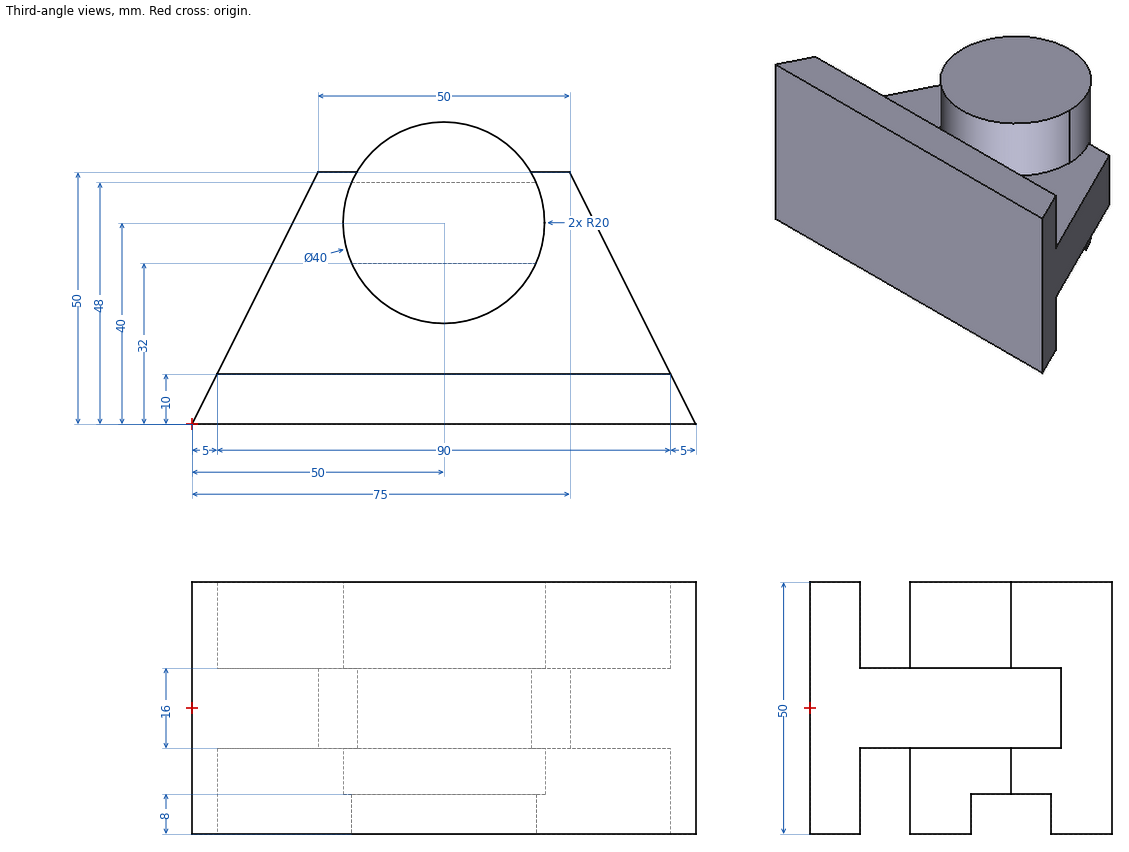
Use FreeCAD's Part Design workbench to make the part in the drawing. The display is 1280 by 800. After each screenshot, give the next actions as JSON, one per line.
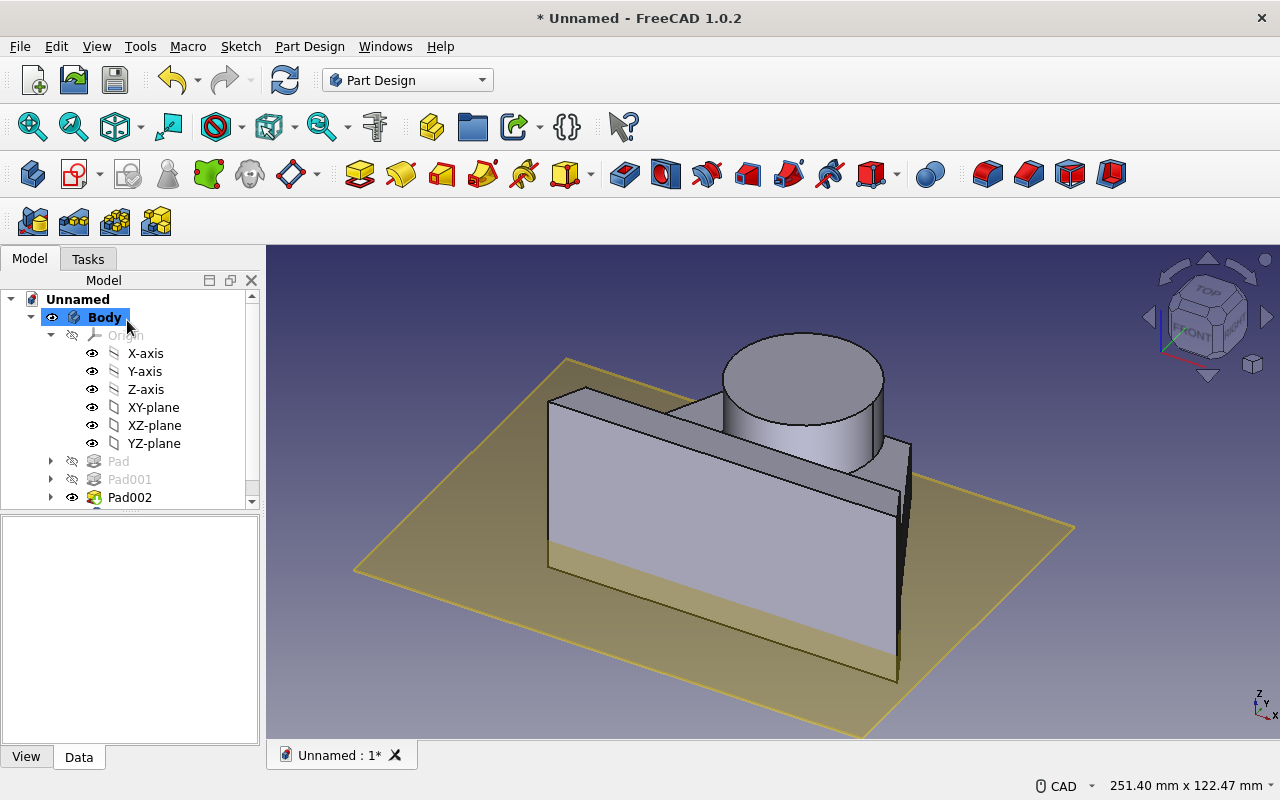
{"action": "scroll", "coordinate": [101, 403], "scroll_direction": "down", "scroll_amount": 3}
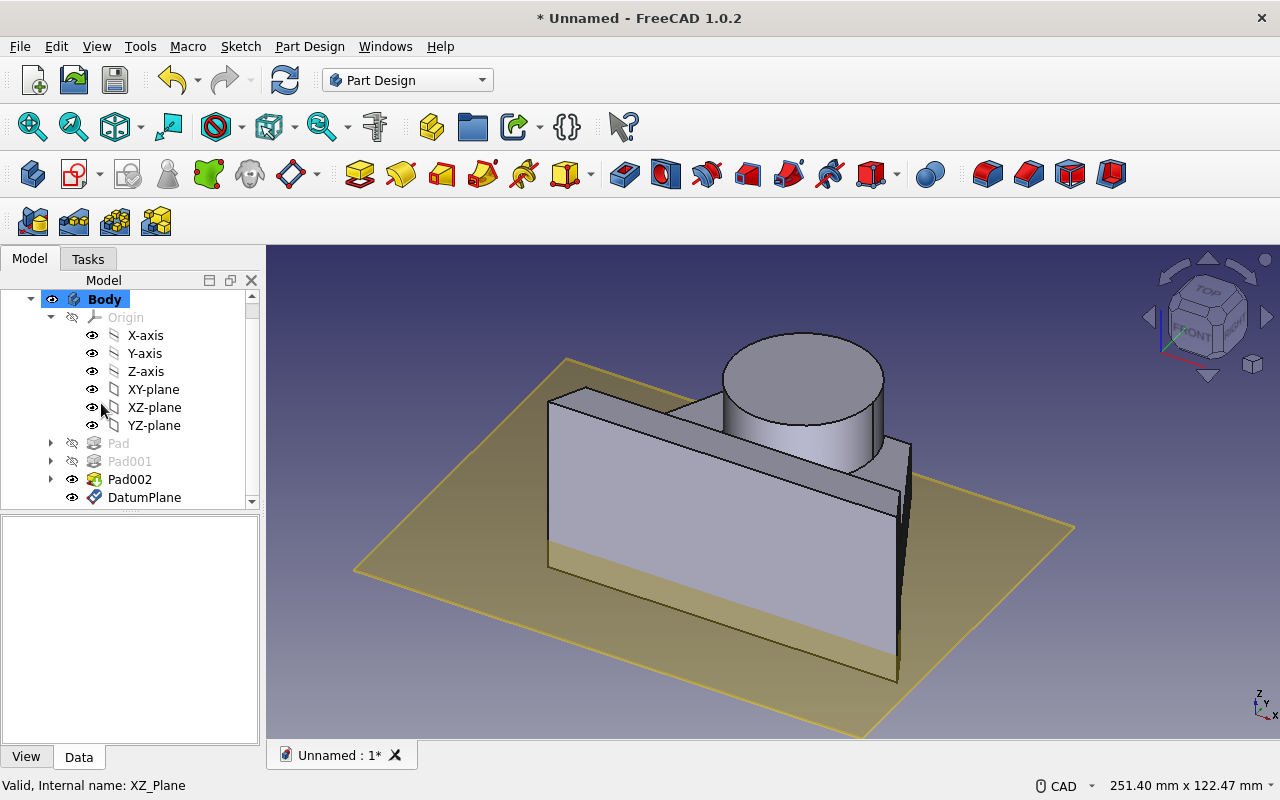
{"action": "left_click", "coordinate": [117, 497]}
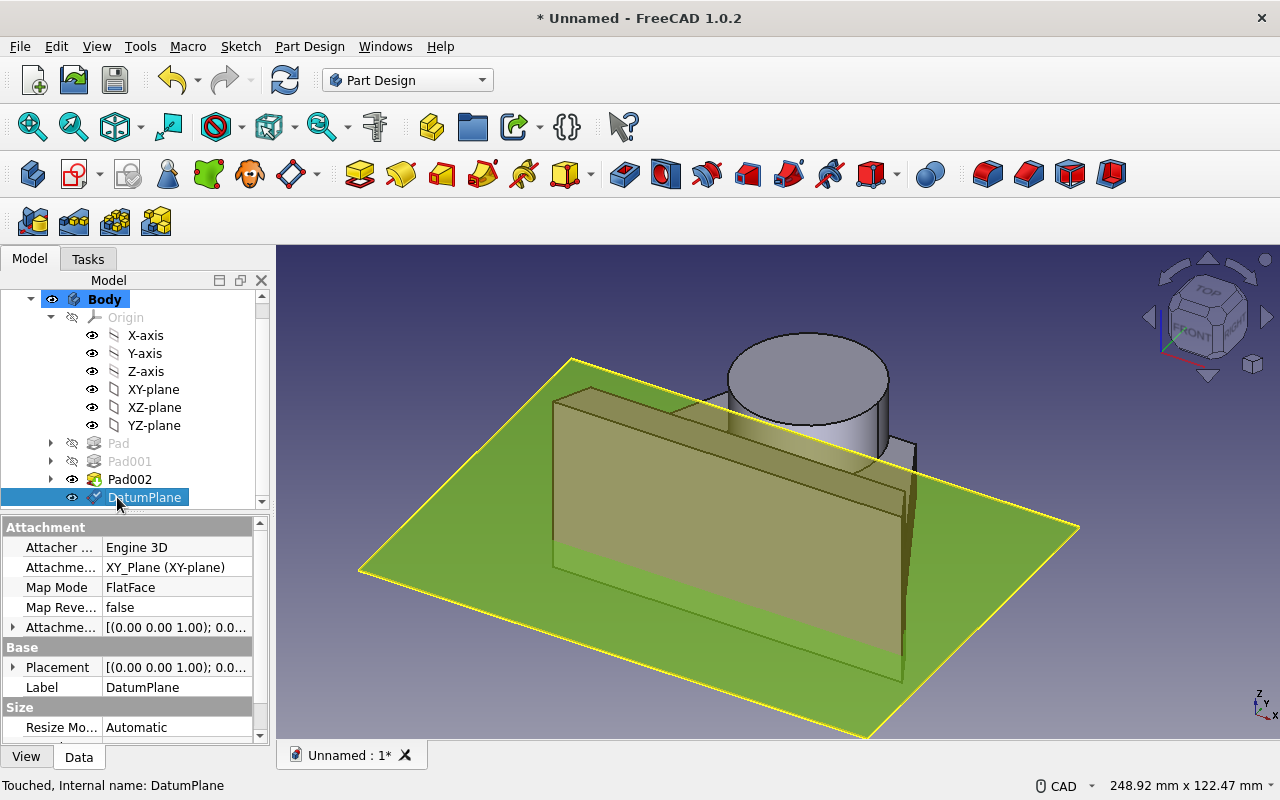
{"action": "left_click", "coordinate": [74, 174]}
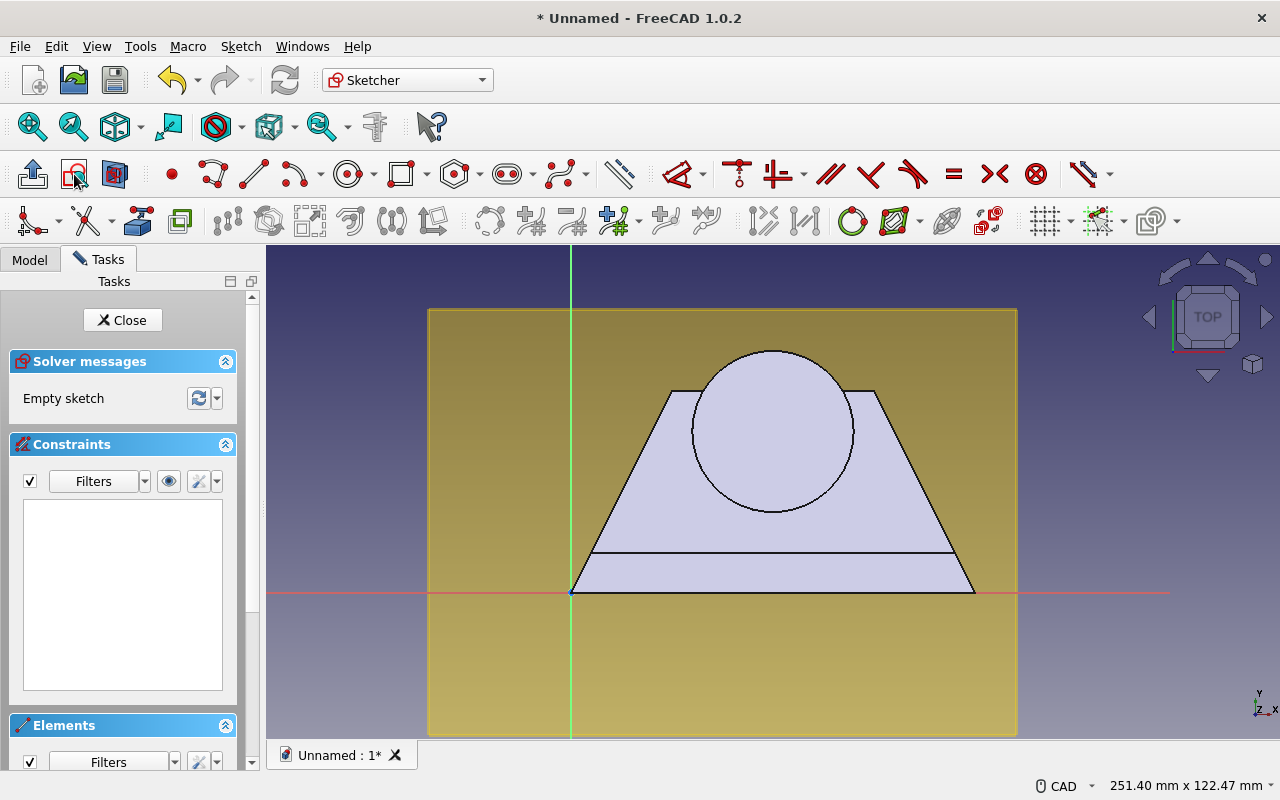
{"action": "left_click", "coordinate": [115, 174]}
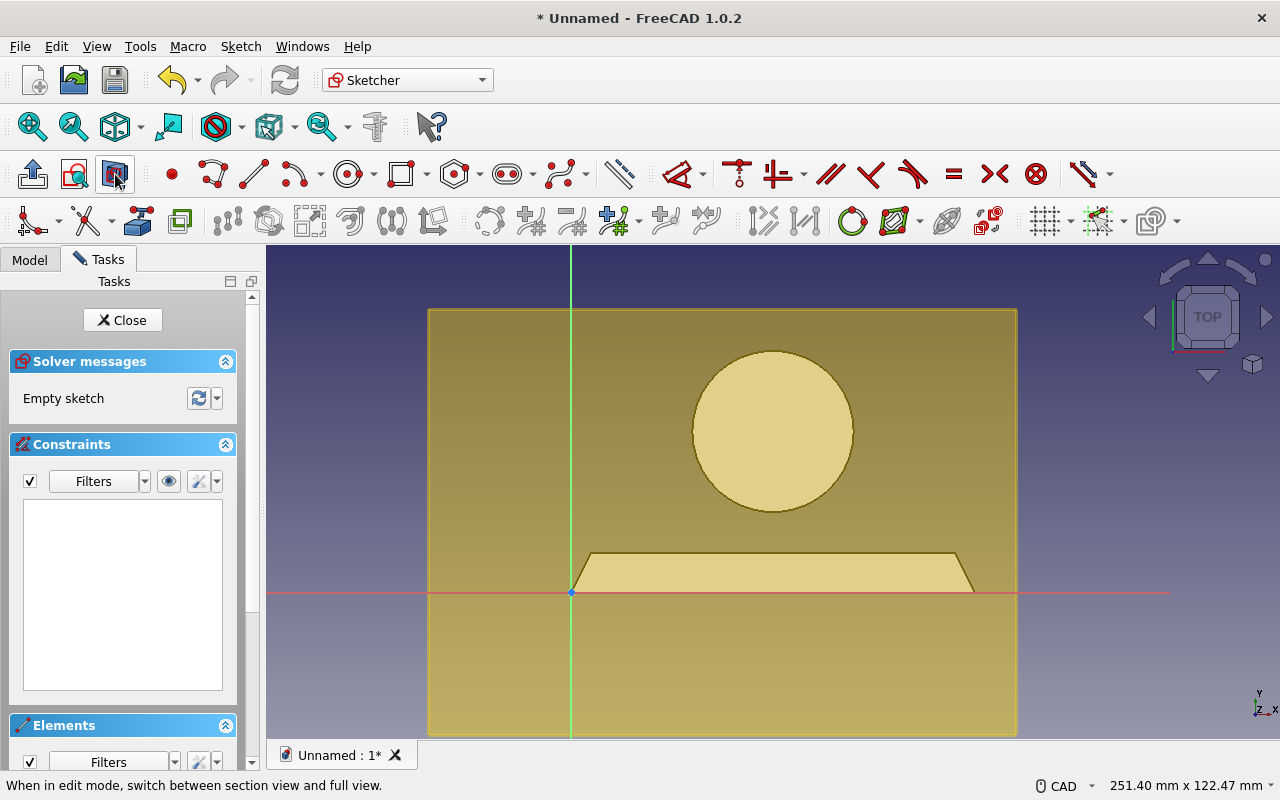
{"action": "scroll", "coordinate": [729, 504], "scroll_direction": "up", "scroll_amount": 2}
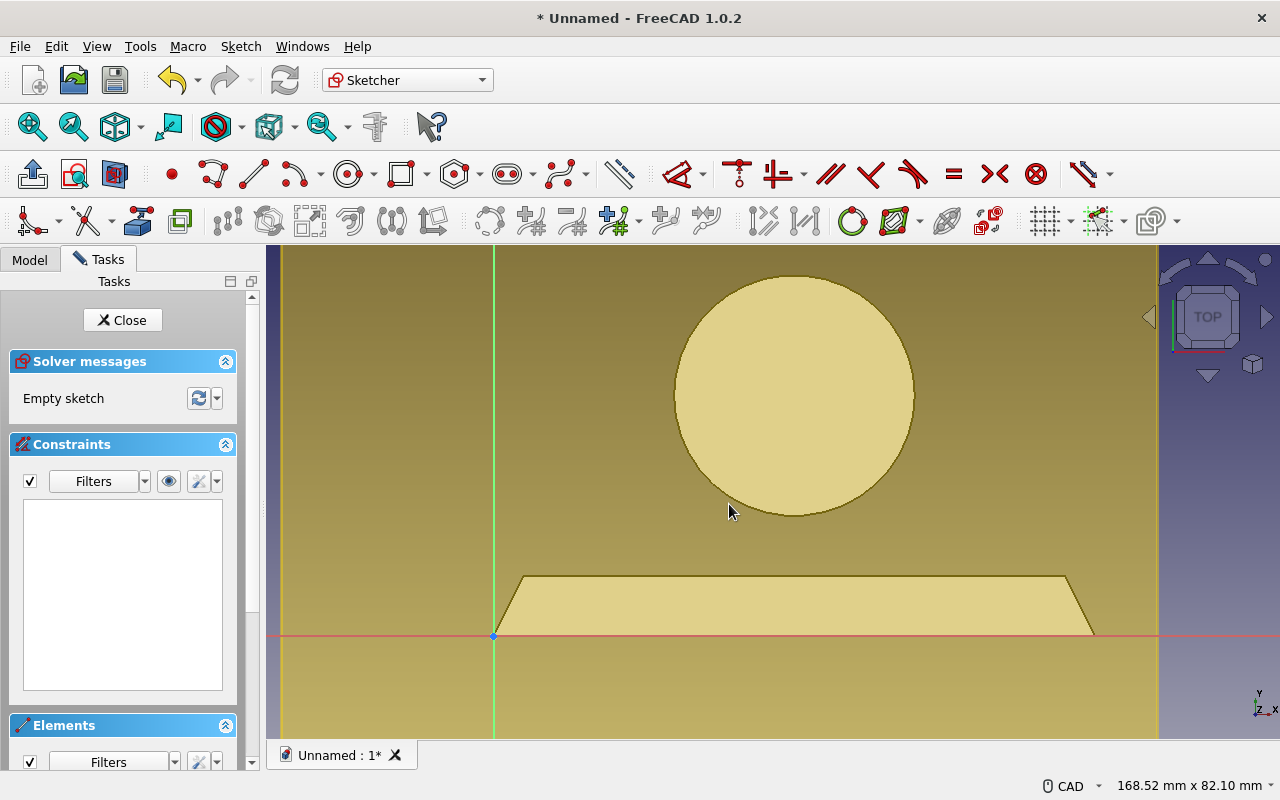
{"action": "left_click", "coordinate": [254, 174]}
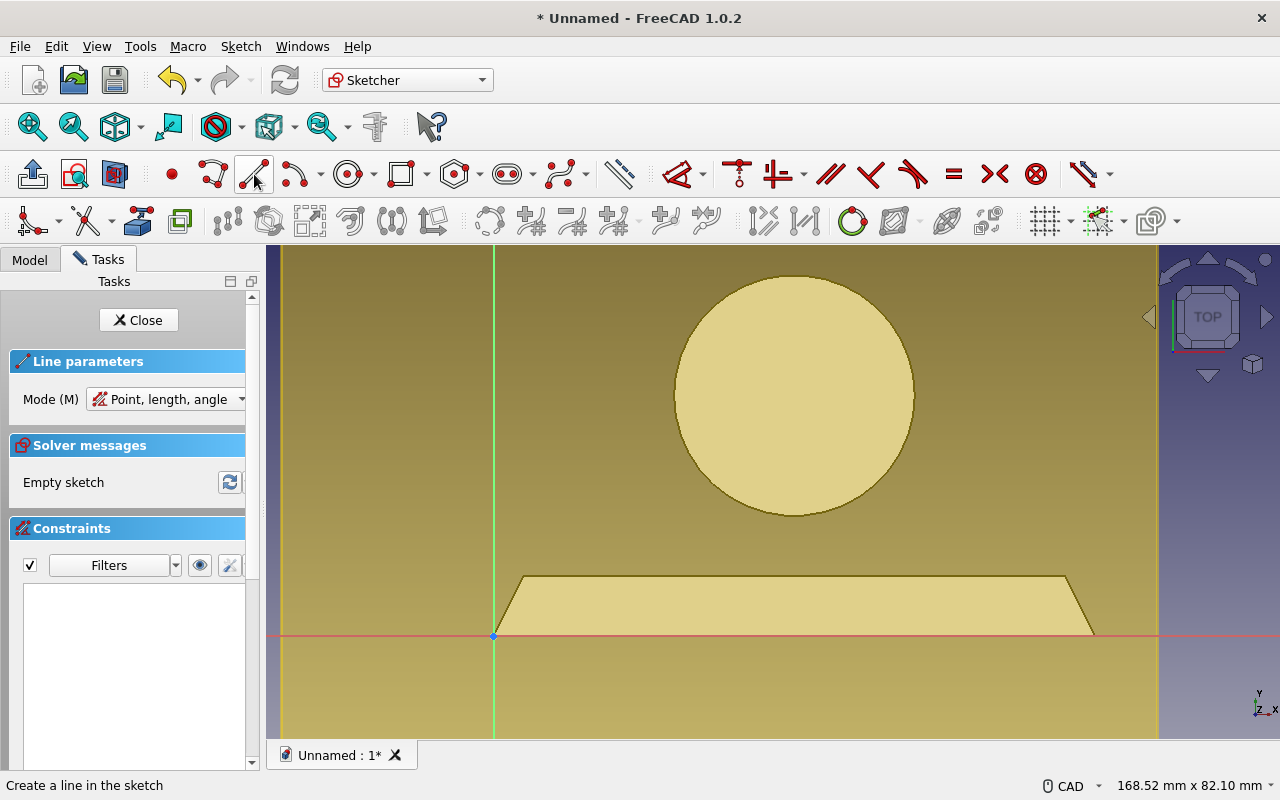
{"action": "left_click", "coordinate": [684, 347]}
{"action": "left_click", "coordinate": [905, 347]}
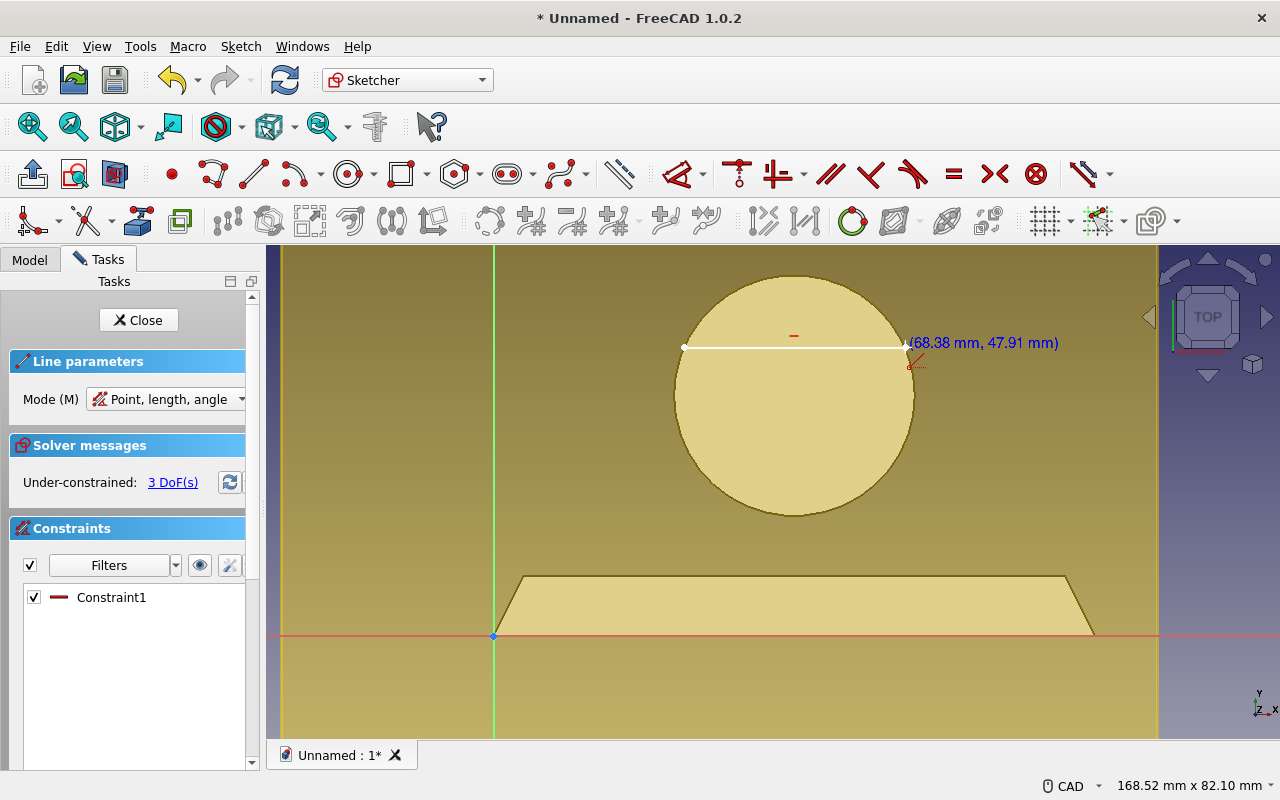
{"action": "left_click", "coordinate": [905, 444]}
{"action": "left_click", "coordinate": [684, 444]}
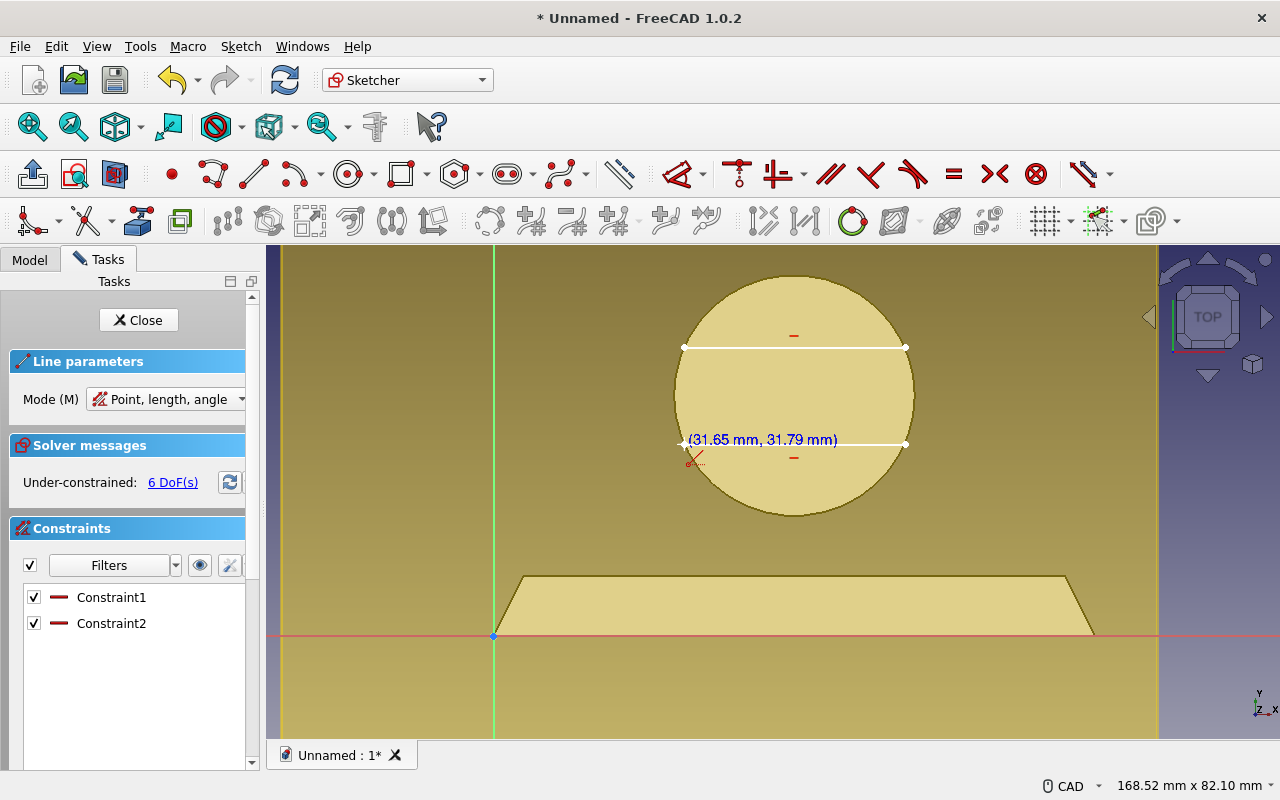
{"action": "key", "text": "g 3 a"}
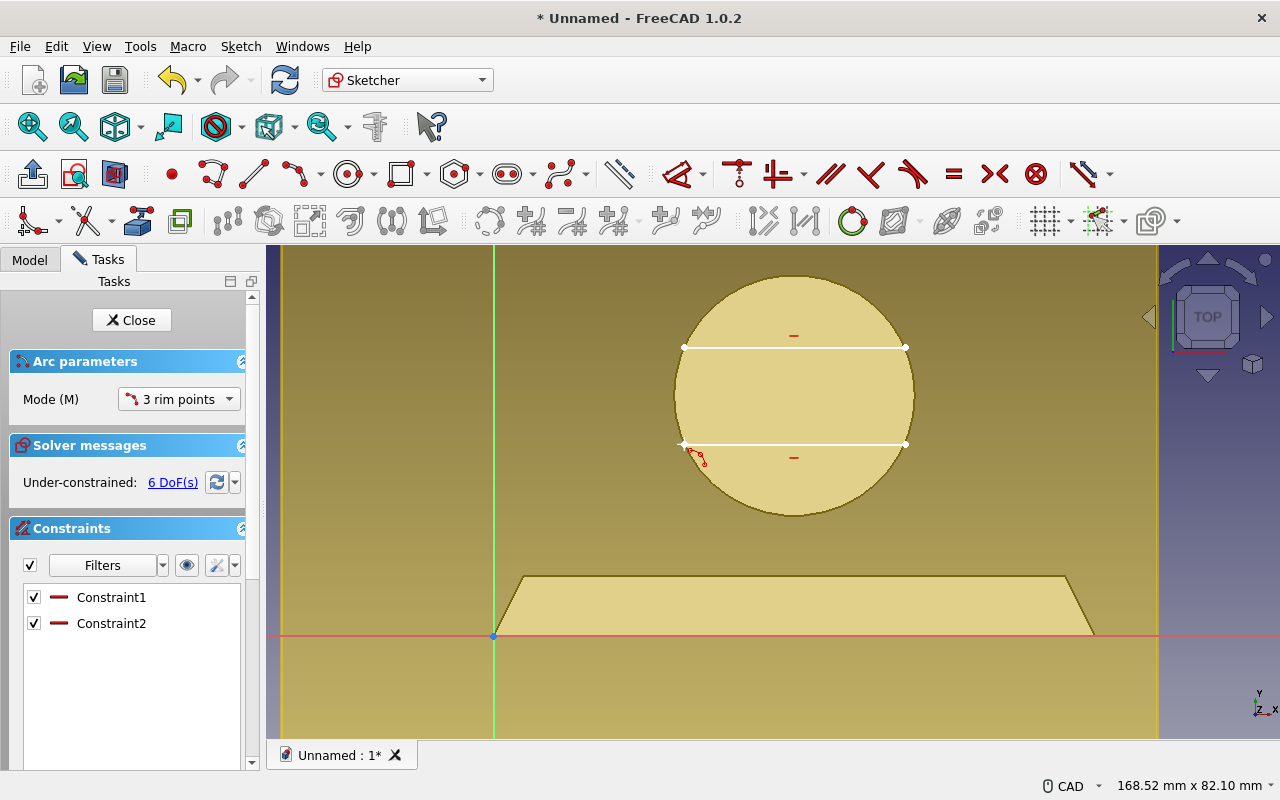
{"action": "left_click", "coordinate": [905, 348]}
{"action": "left_click", "coordinate": [905, 445]}